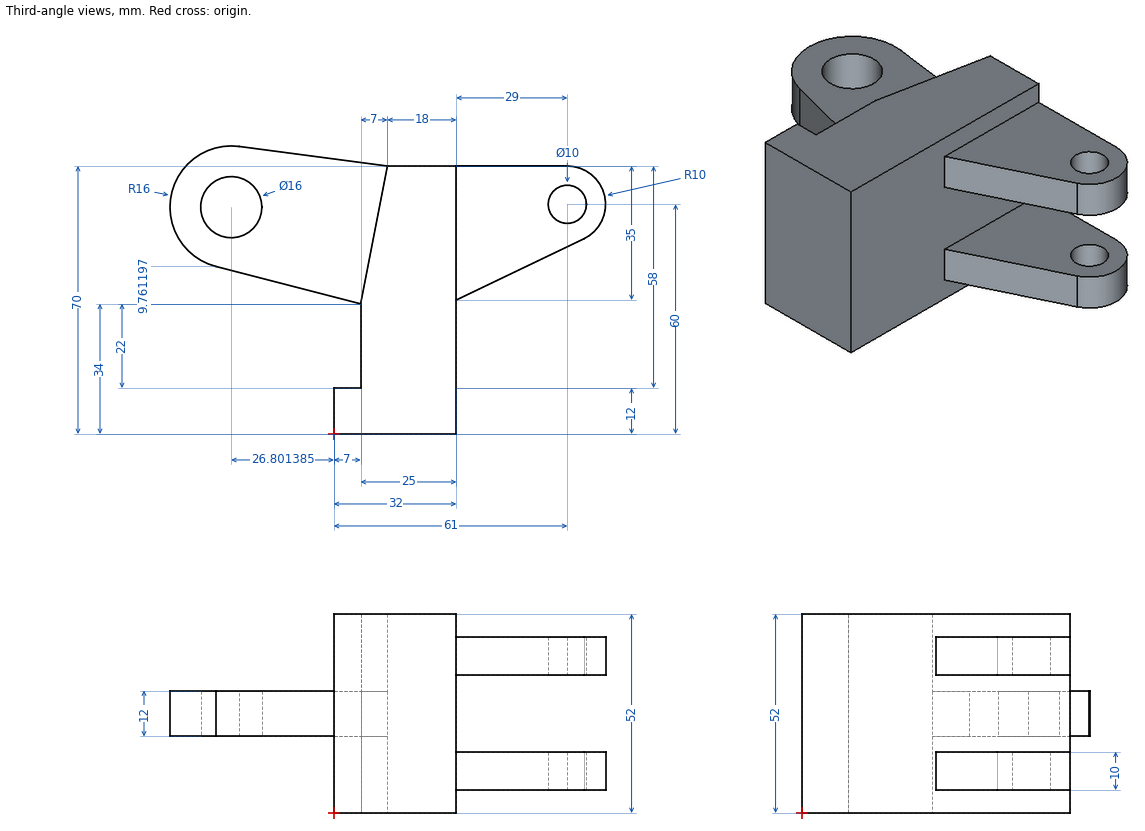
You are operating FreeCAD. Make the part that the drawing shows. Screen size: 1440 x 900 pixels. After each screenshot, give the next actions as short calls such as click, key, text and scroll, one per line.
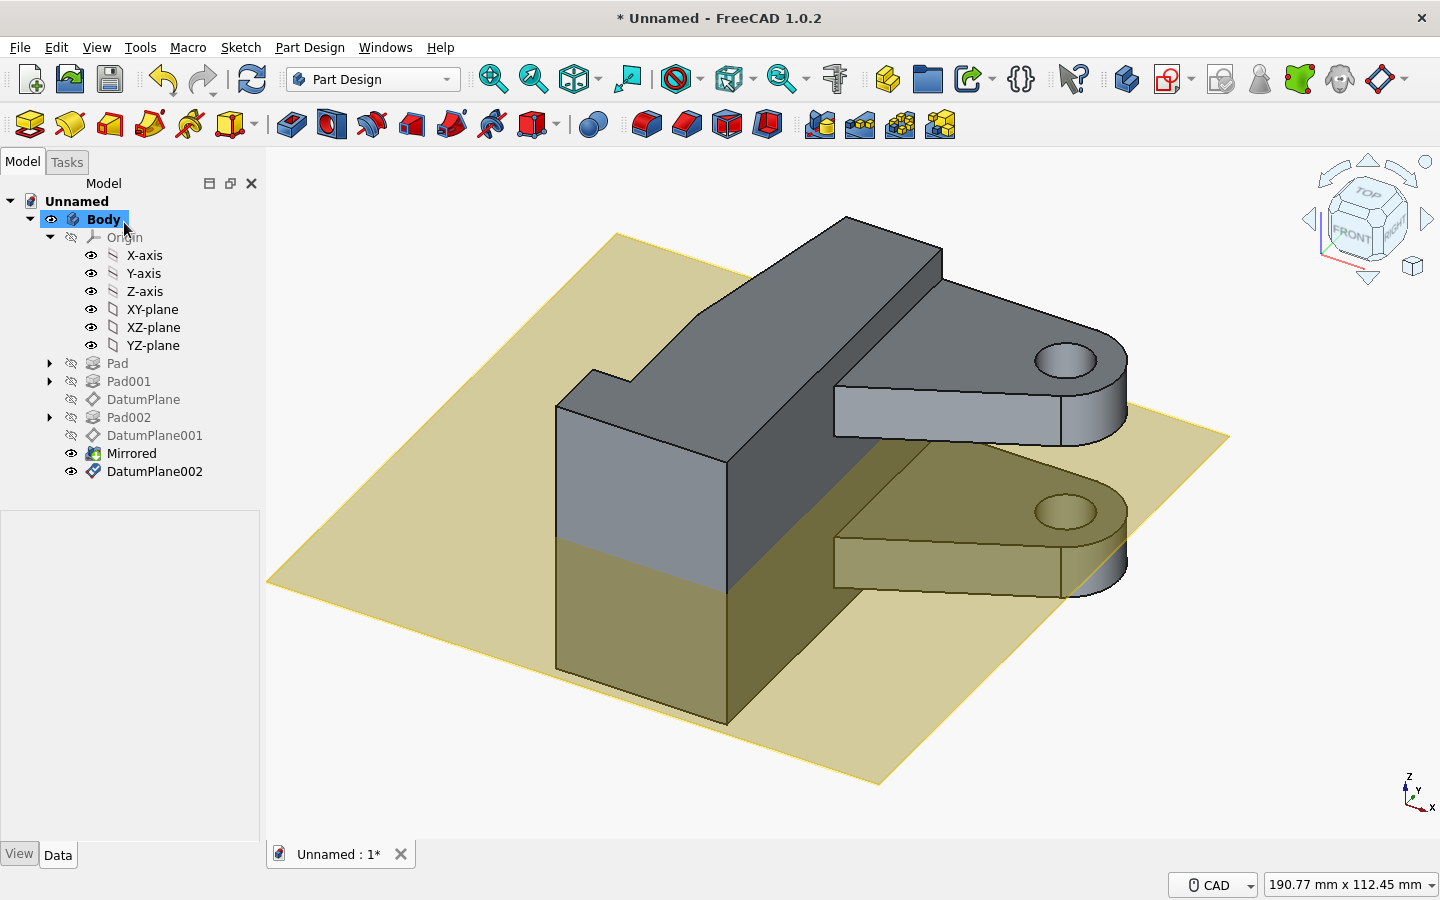
click(116, 471)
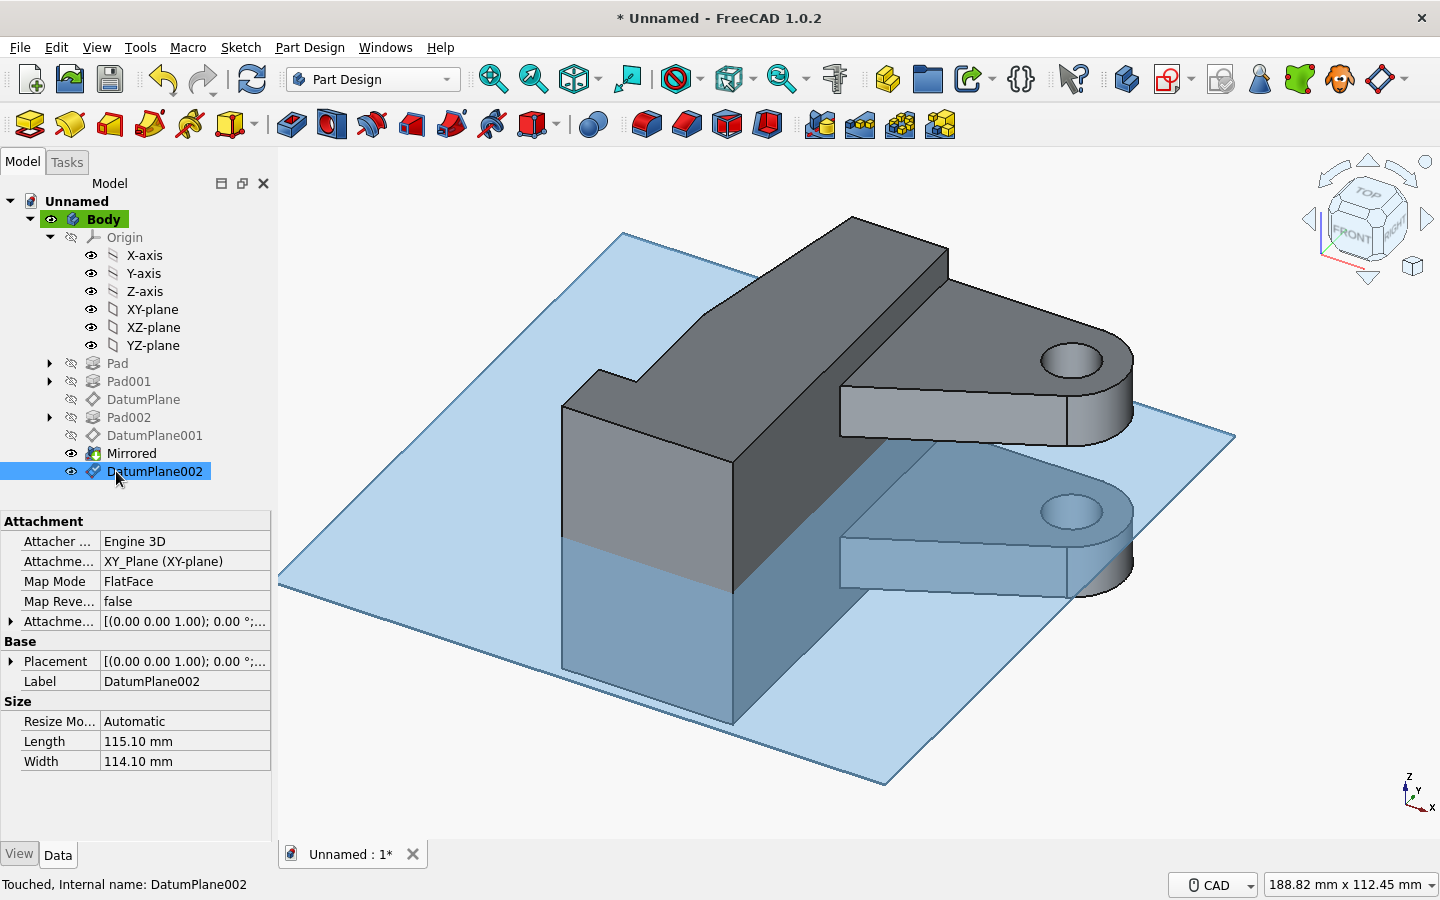
click(1168, 80)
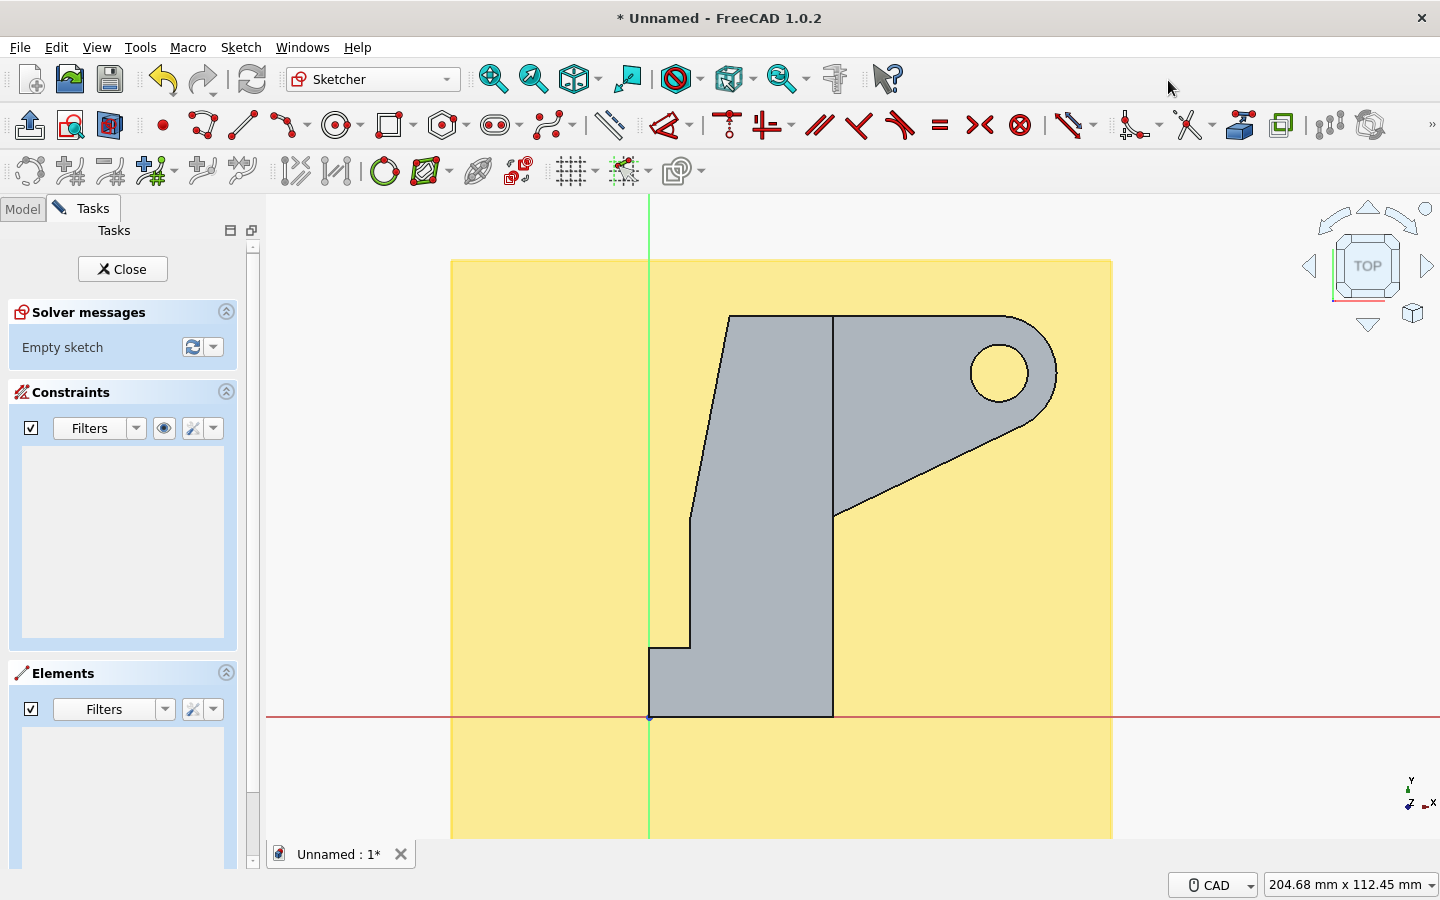
key(q)
key(s)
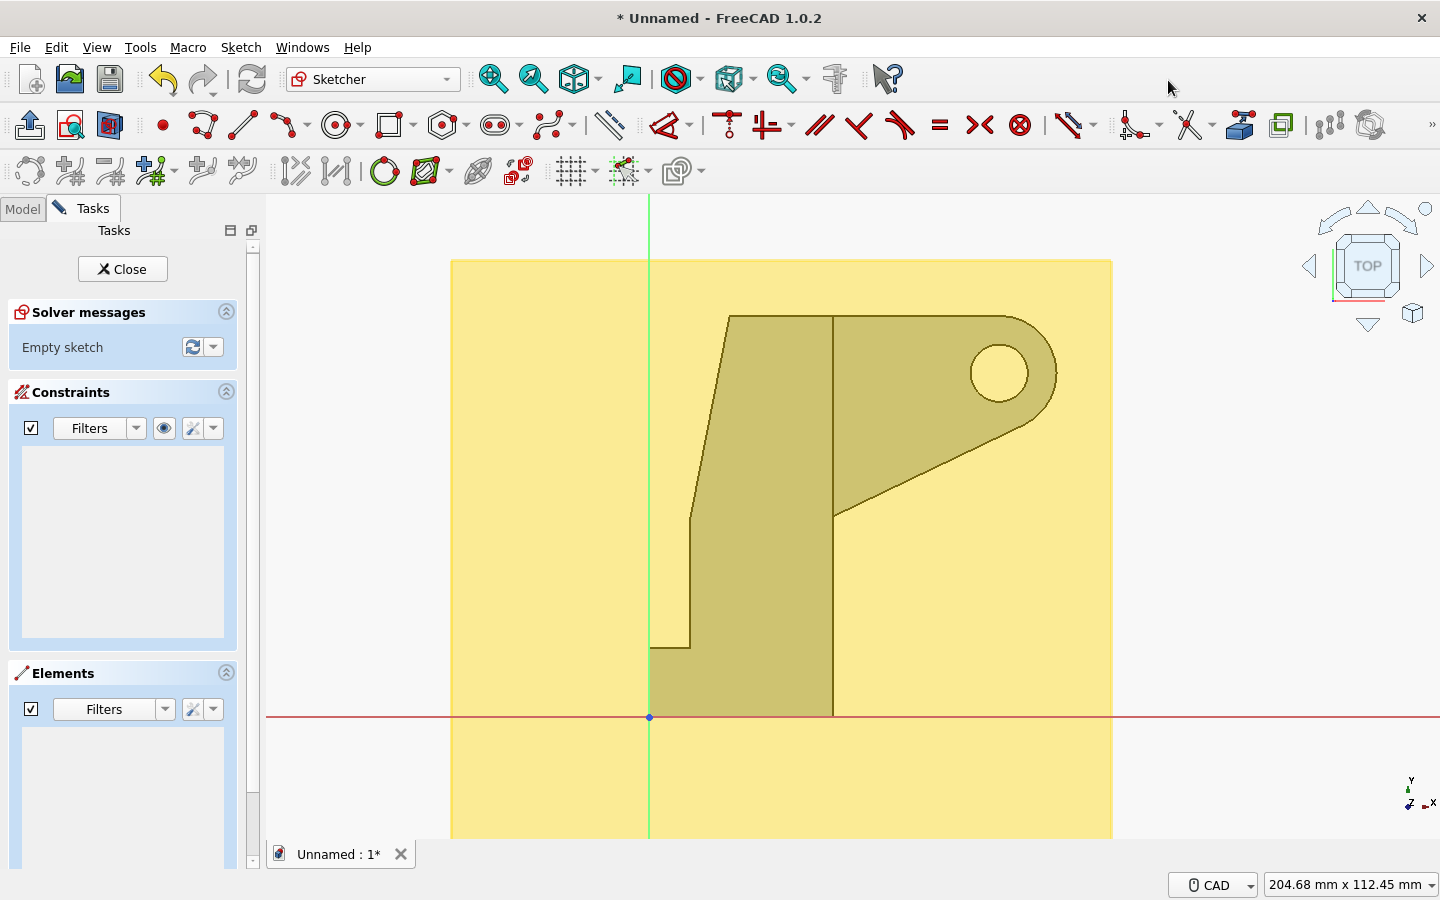
click(204, 126)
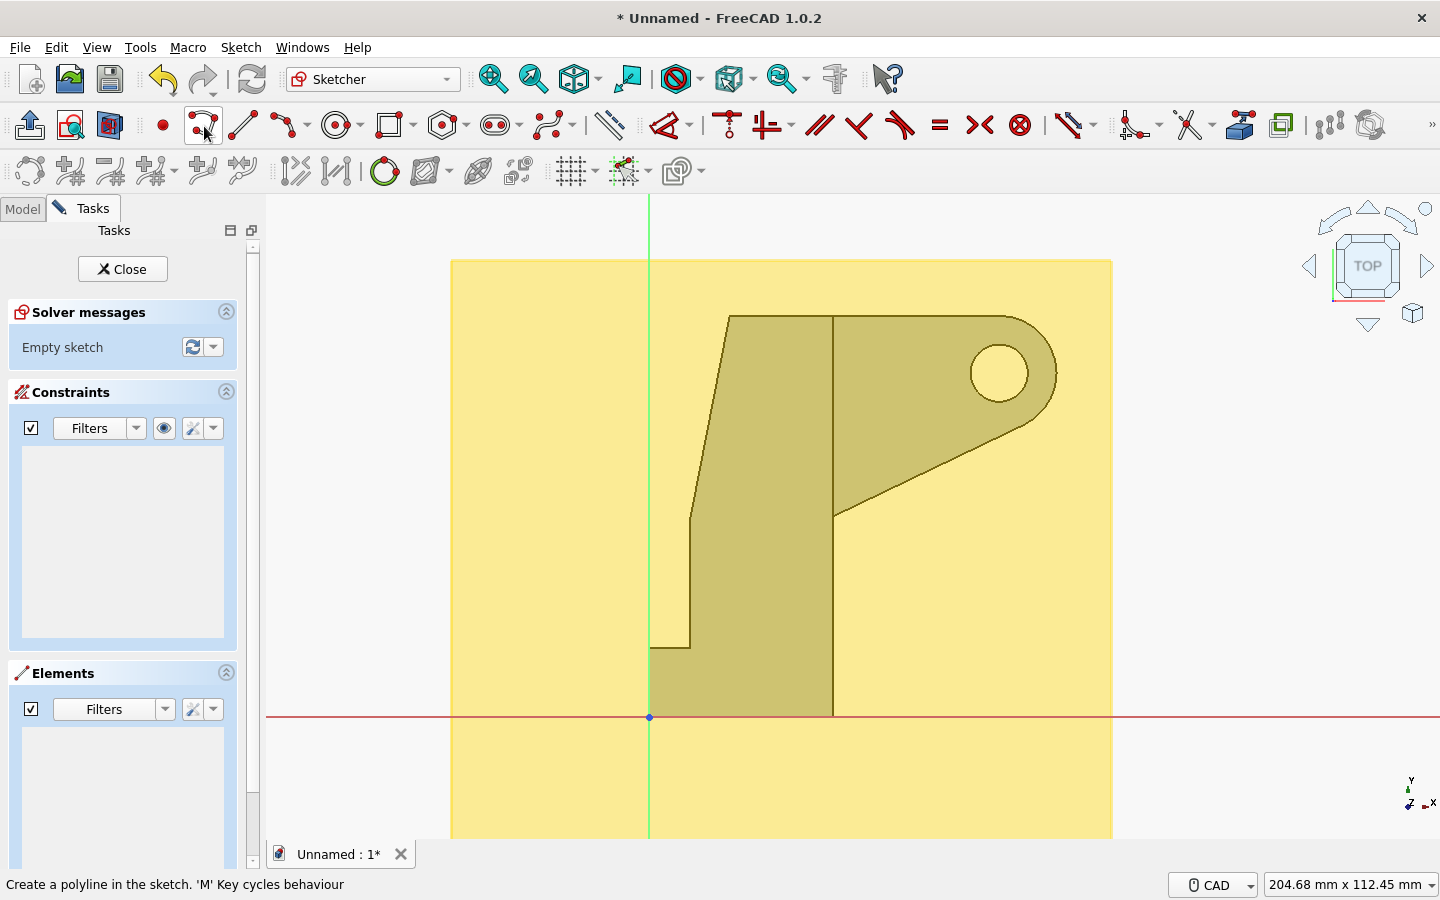
click(473, 466)
click(690, 522)
click(730, 316)
click(508, 286)
right_click(508, 286)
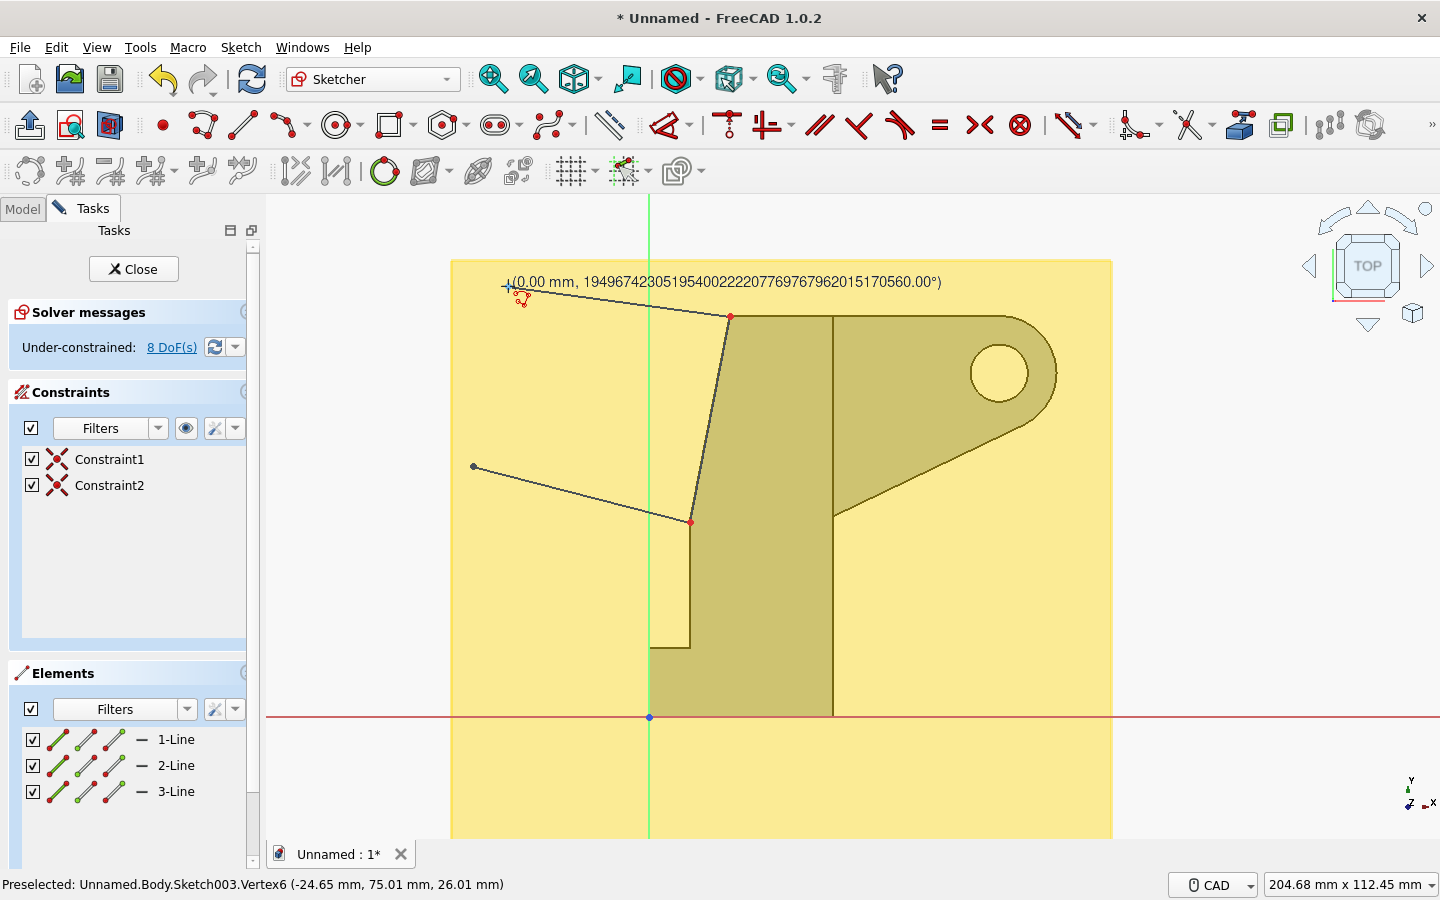
click(284, 126)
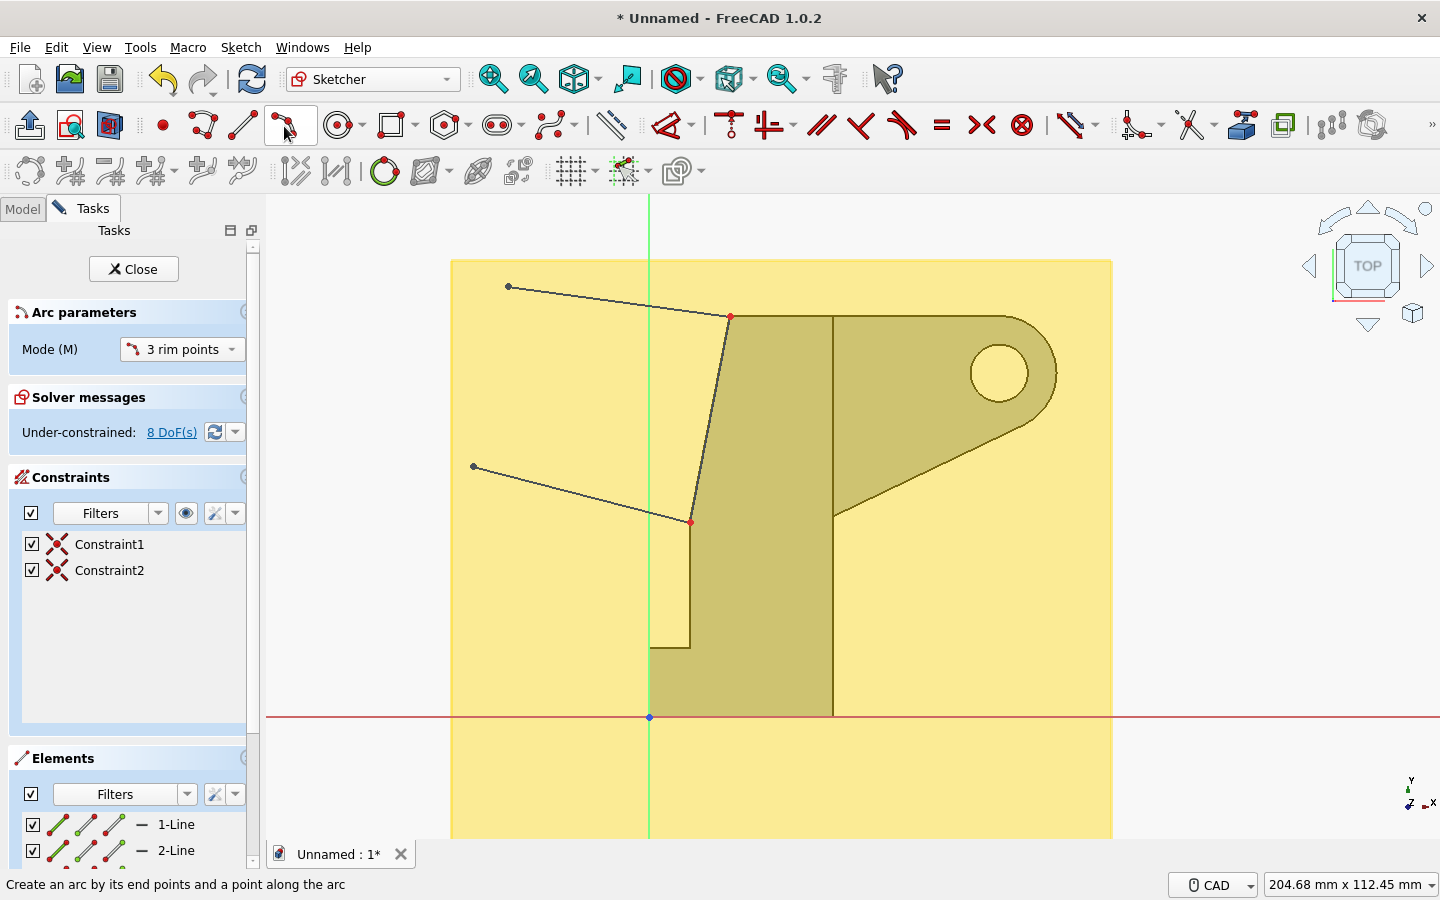
click(508, 287)
click(473, 467)
click(406, 360)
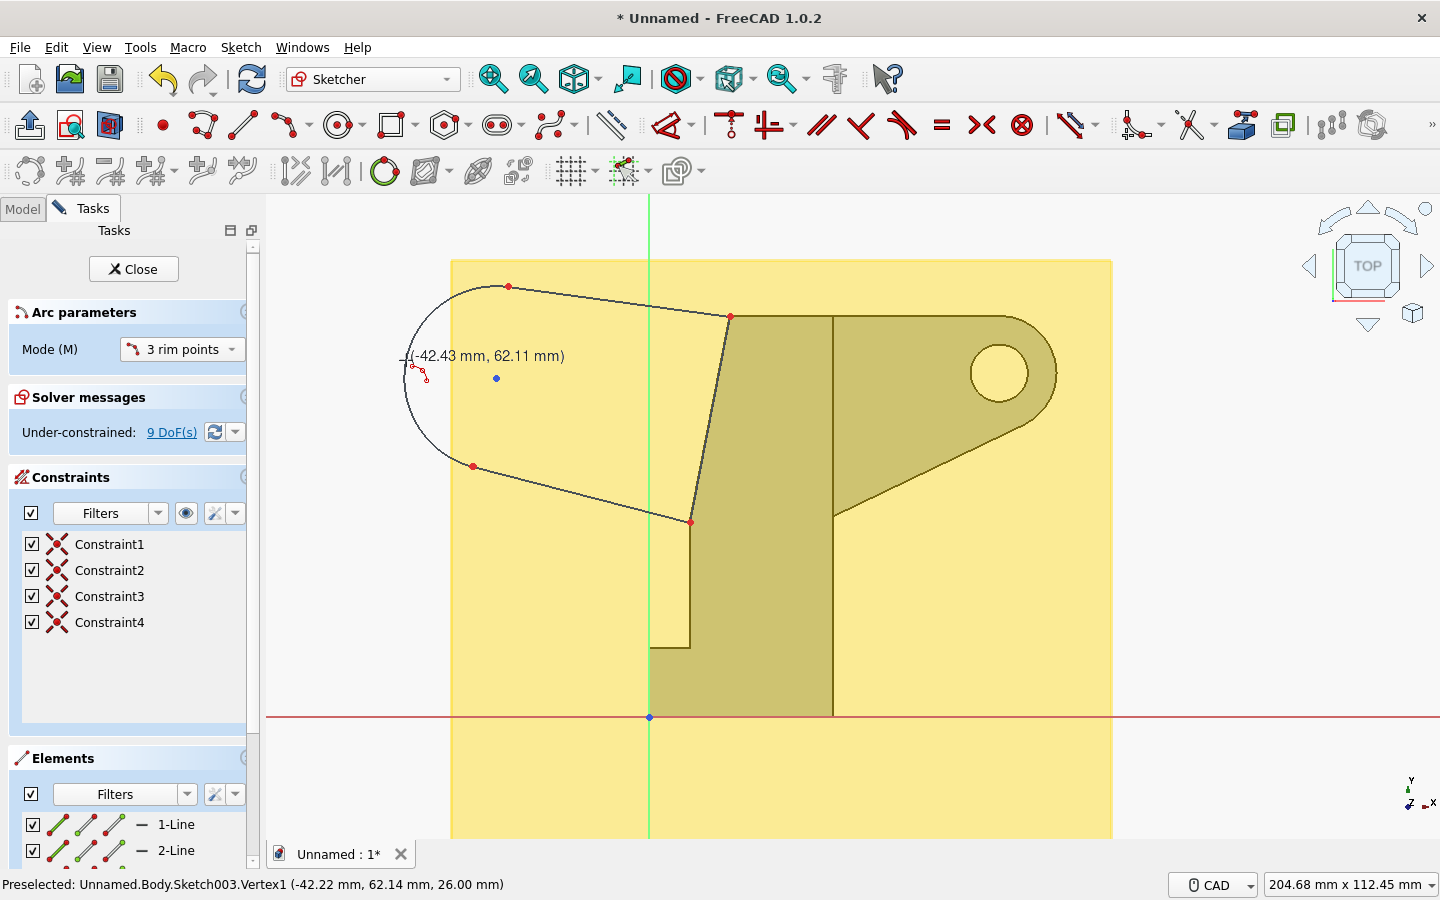
click(338, 126)